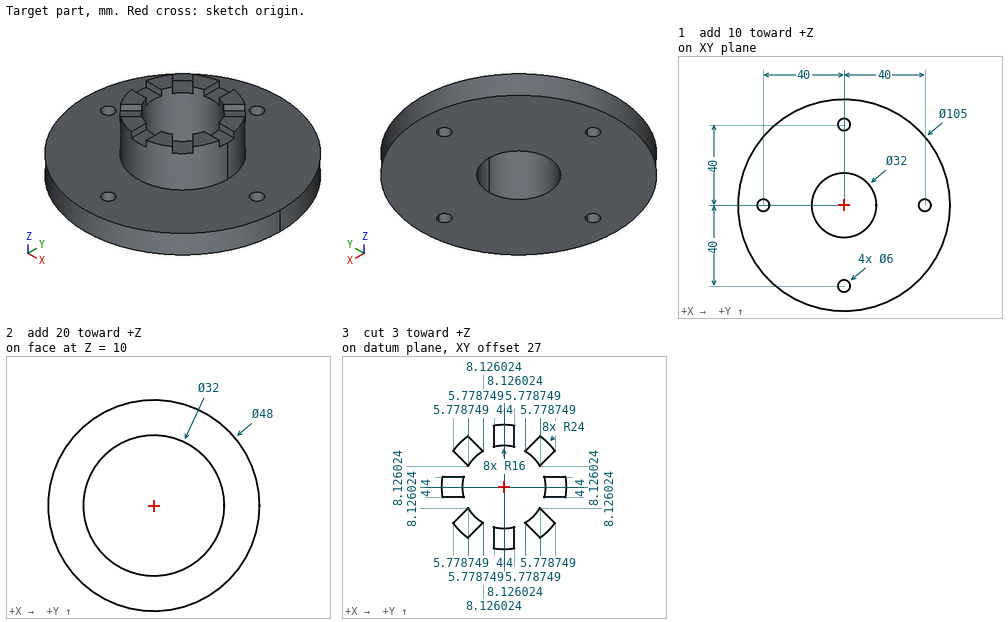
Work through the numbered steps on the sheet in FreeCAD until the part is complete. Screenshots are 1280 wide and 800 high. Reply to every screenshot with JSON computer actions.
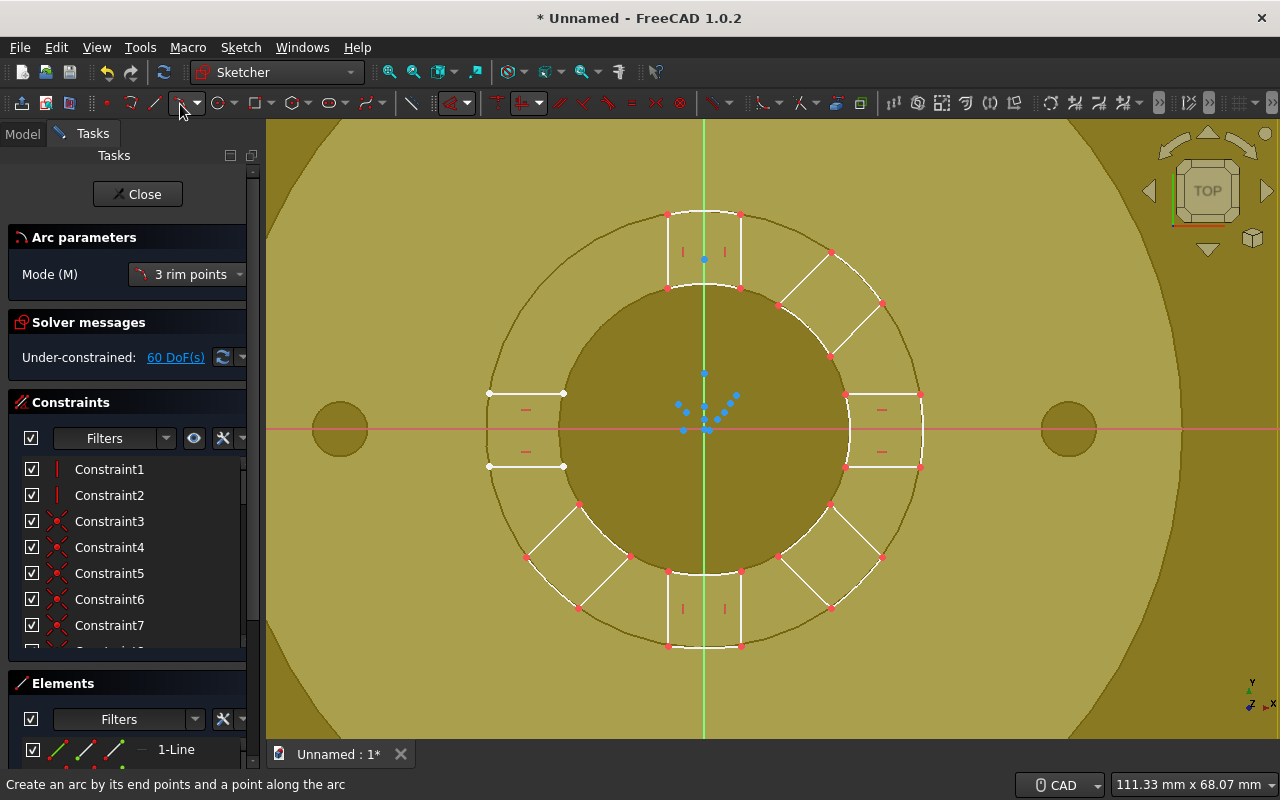
{"action": "left_click", "coordinate": [563, 467]}
{"action": "left_click", "coordinate": [563, 394]}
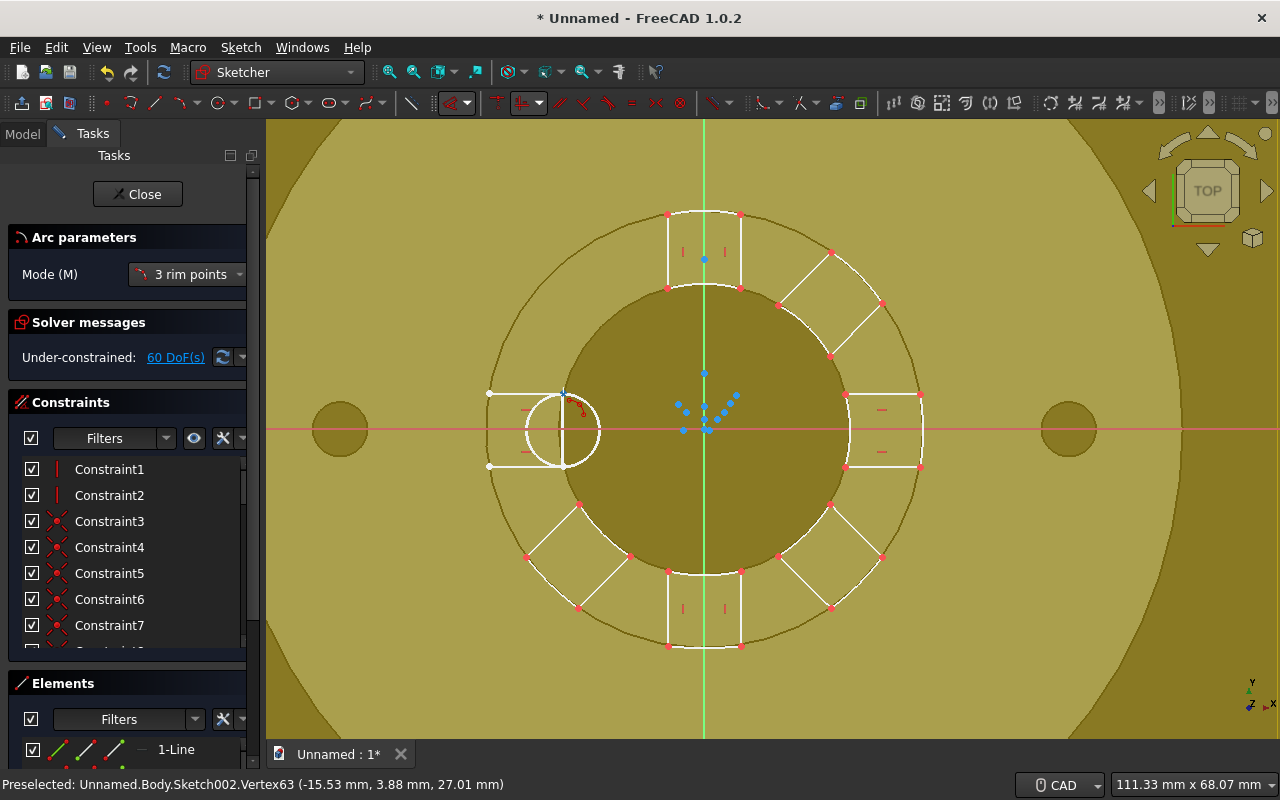
{"action": "scroll", "coordinate": [559, 422], "scroll_direction": "up", "scroll_amount": 7}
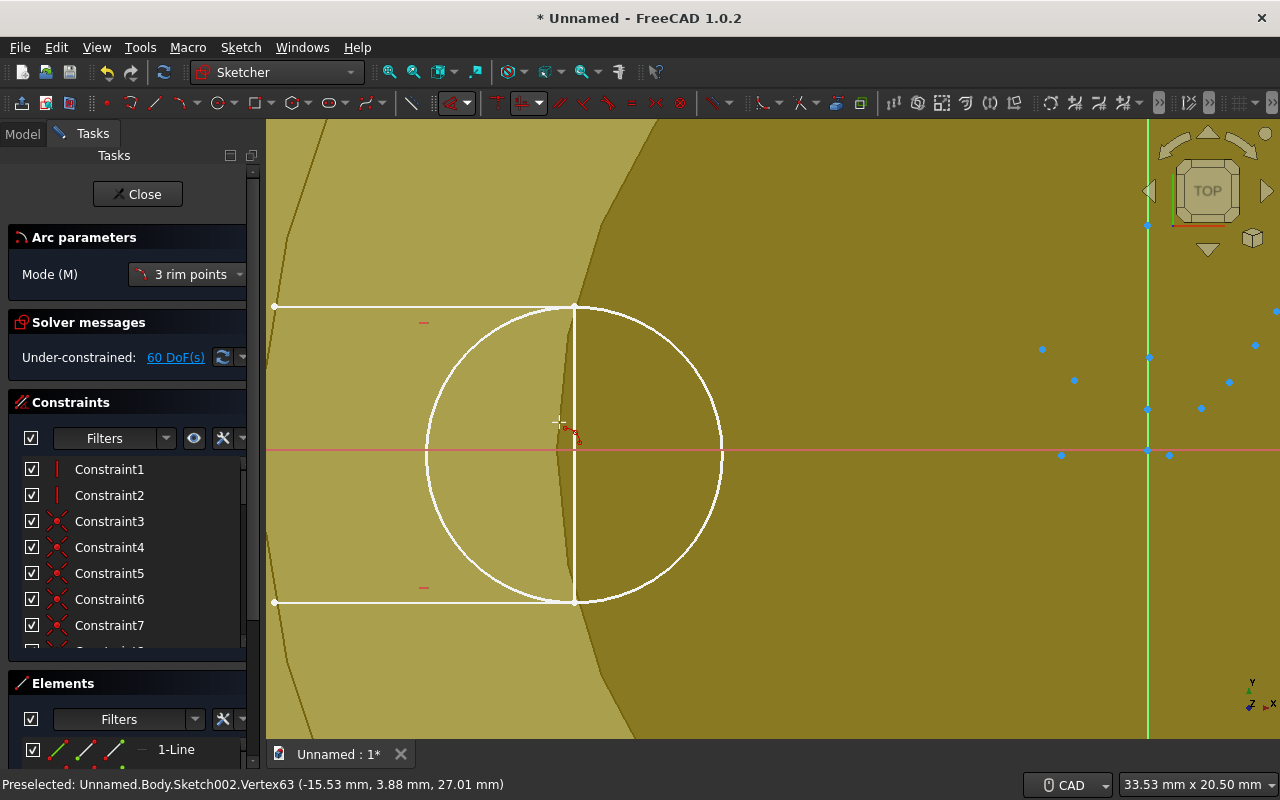
{"action": "left_click", "coordinate": [558, 420]}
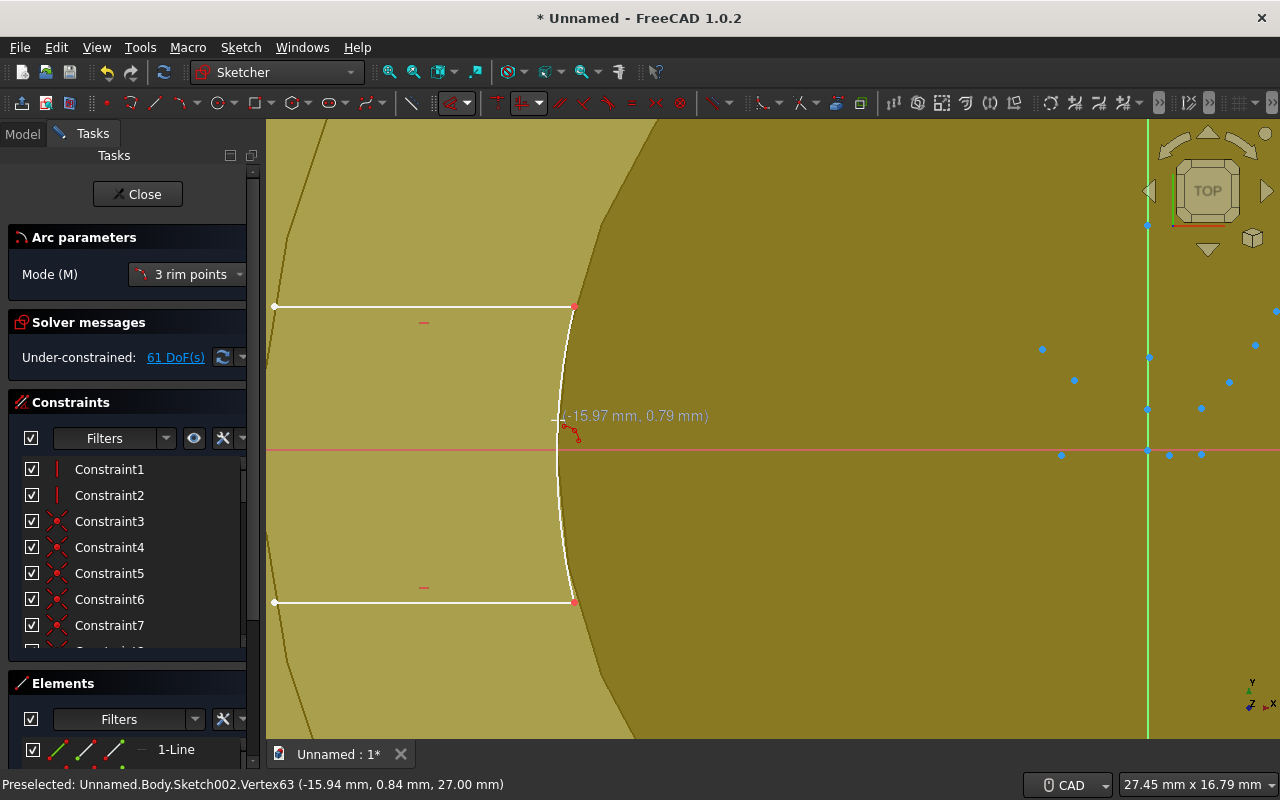
{"action": "scroll", "coordinate": [559, 422], "scroll_direction": "down", "scroll_amount": 7}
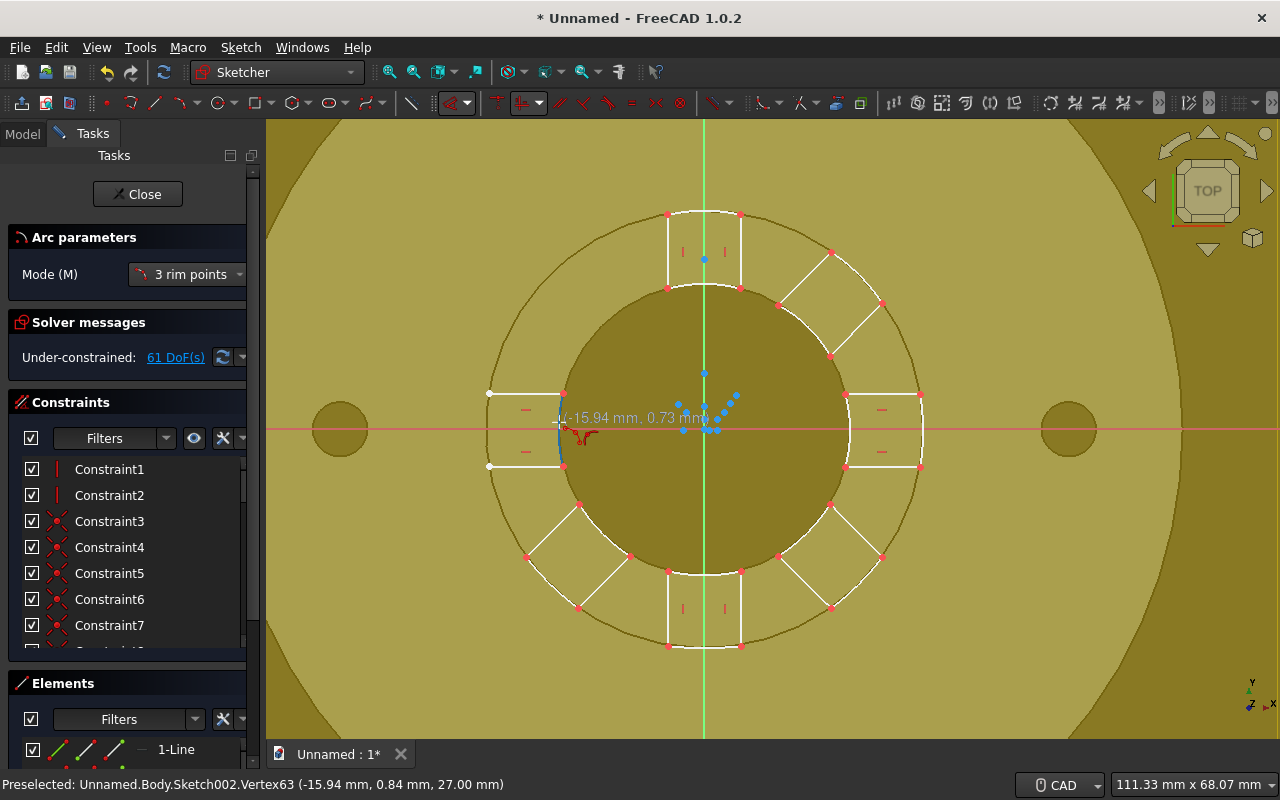
{"action": "left_click", "coordinate": [489, 394]}
{"action": "left_click", "coordinate": [489, 467]}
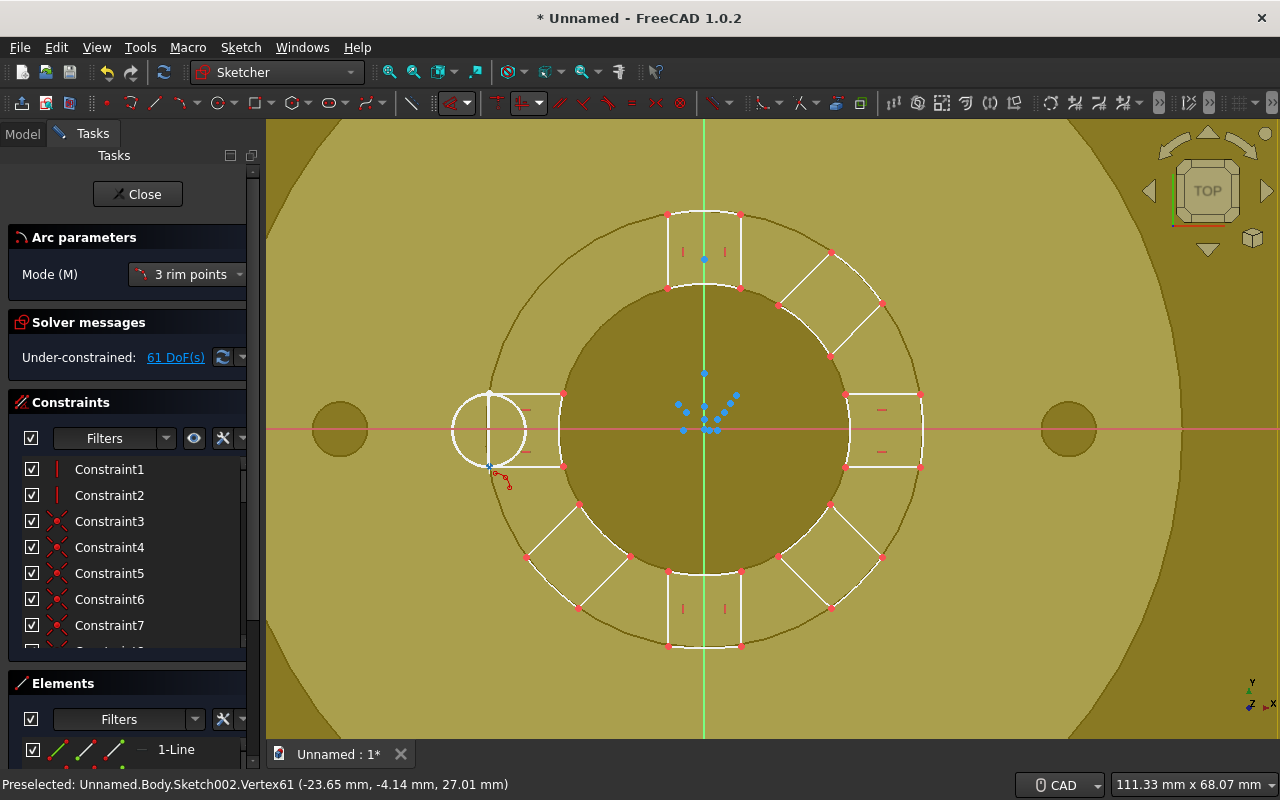
{"action": "scroll", "coordinate": [486, 422], "scroll_direction": "up", "scroll_amount": 9}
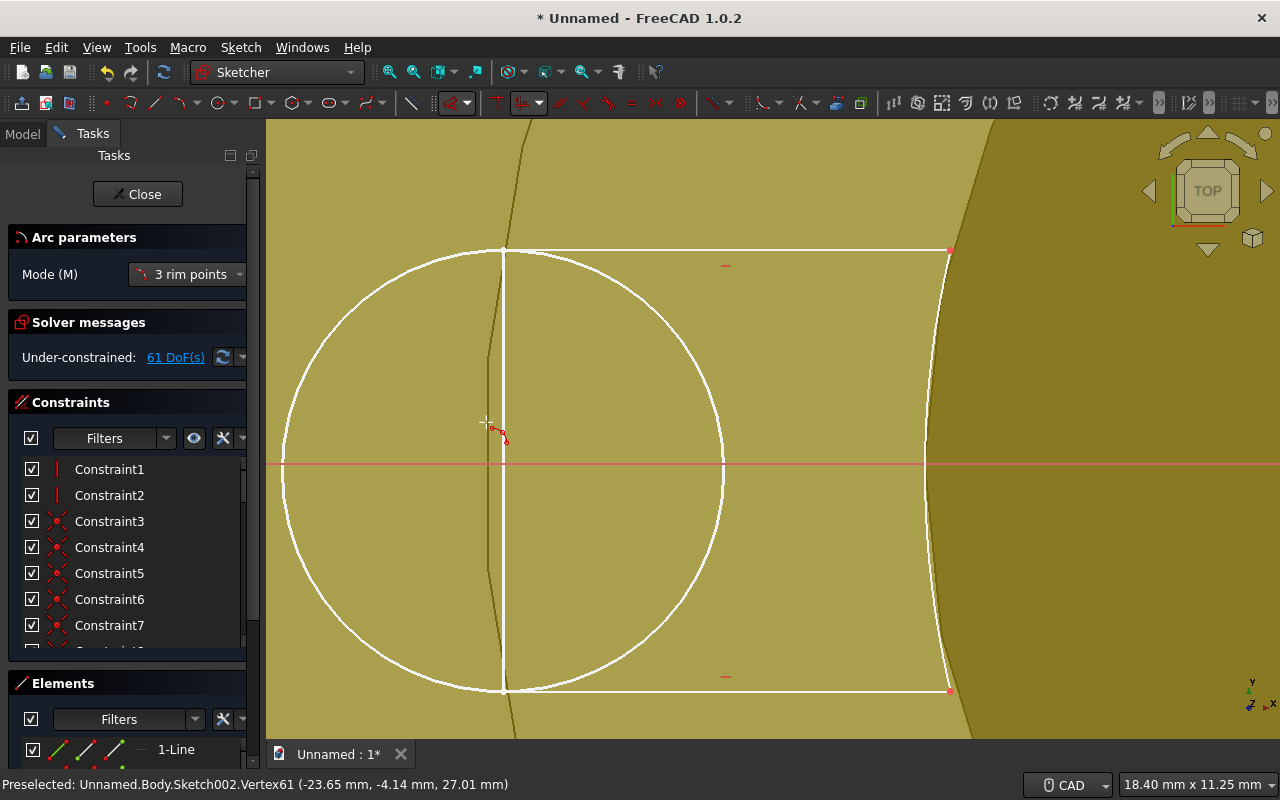
{"action": "left_click", "coordinate": [485, 419]}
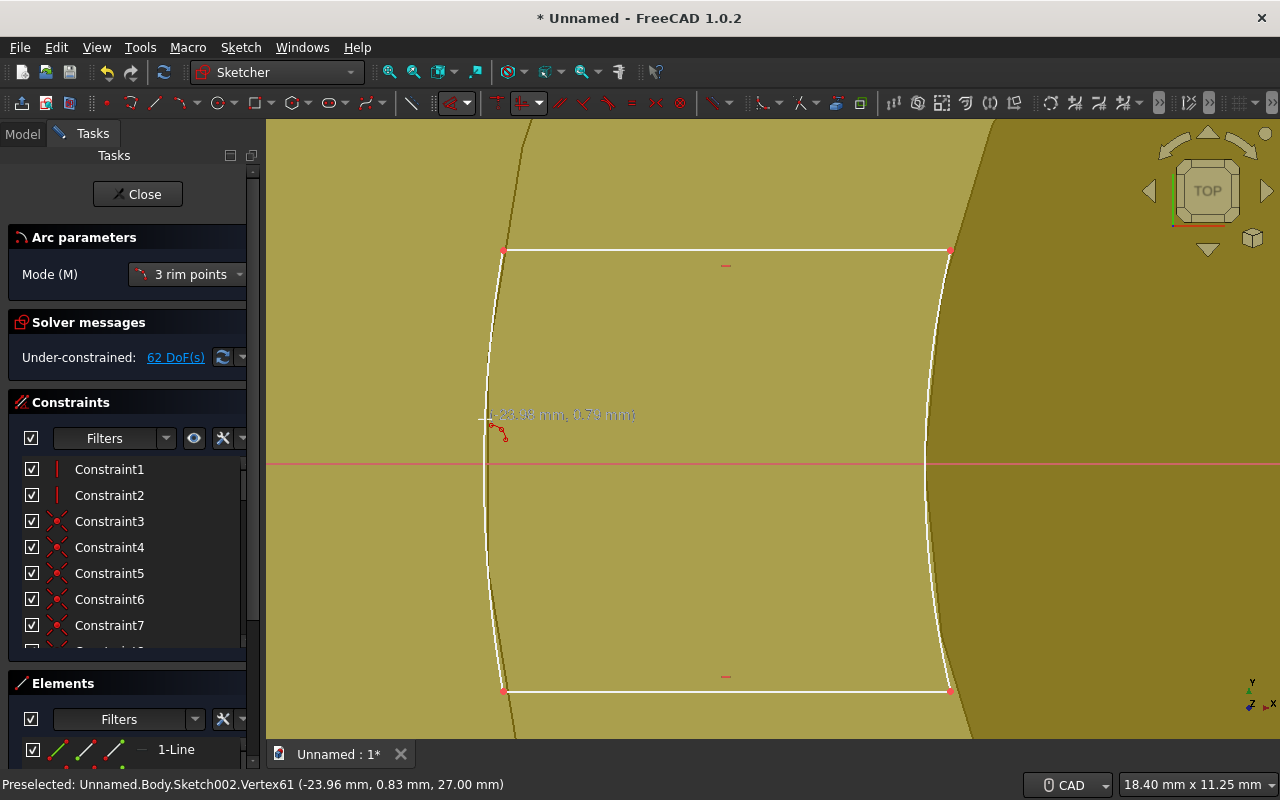
{"action": "left_click", "coordinate": [156, 104]}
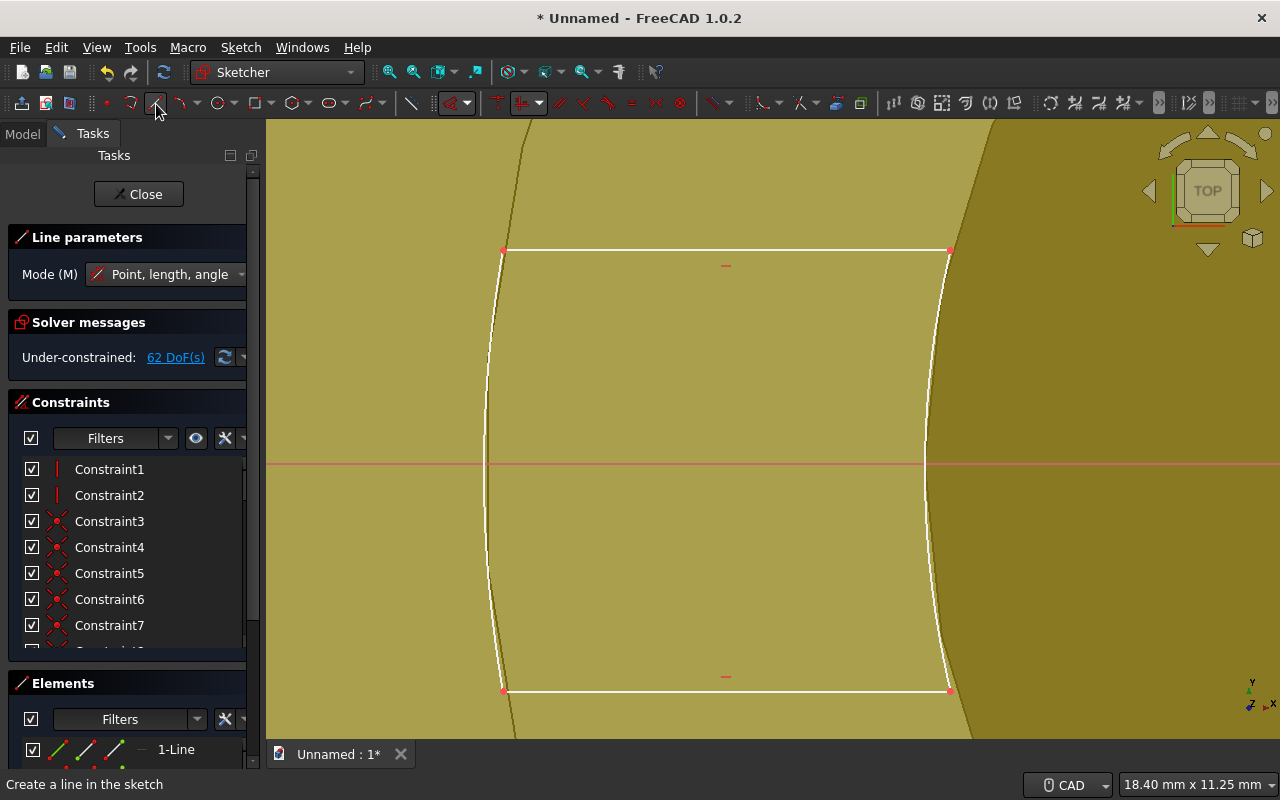
{"action": "scroll", "coordinate": [486, 422], "scroll_direction": "down", "scroll_amount": 9}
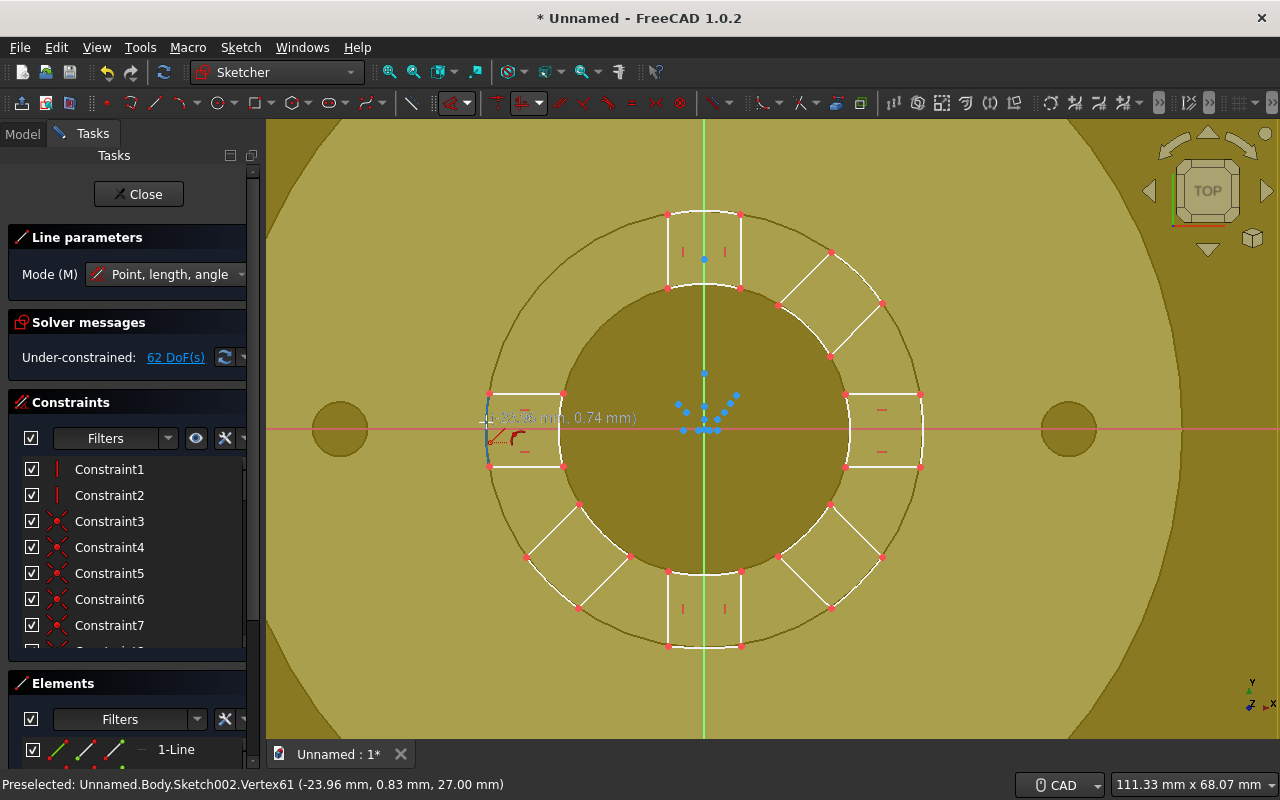
{"action": "left_click", "coordinate": [526, 303]}
{"action": "left_click", "coordinate": [579, 355]}